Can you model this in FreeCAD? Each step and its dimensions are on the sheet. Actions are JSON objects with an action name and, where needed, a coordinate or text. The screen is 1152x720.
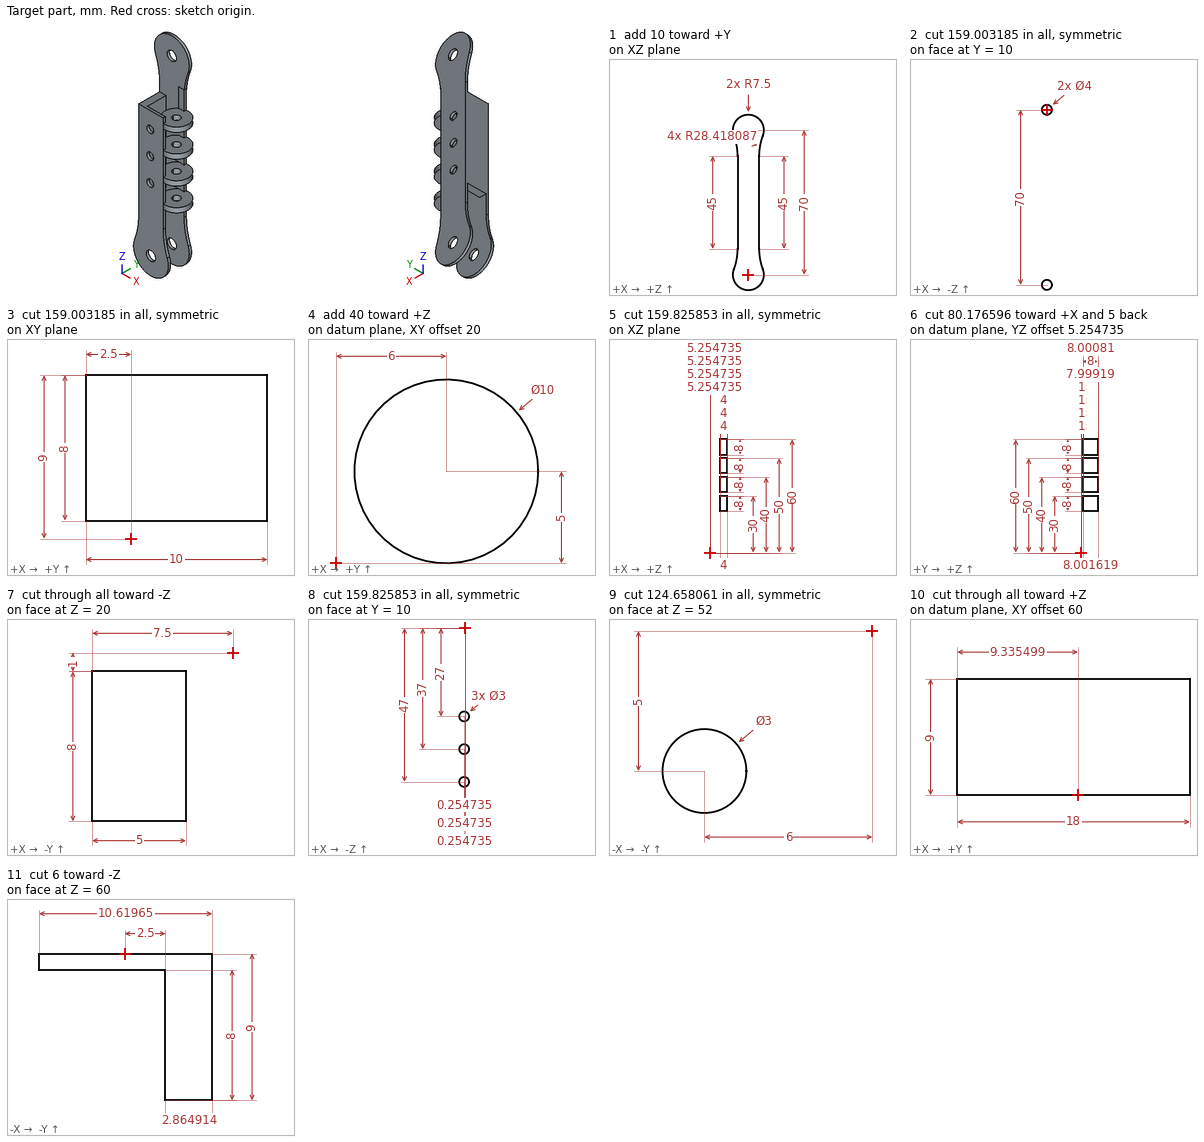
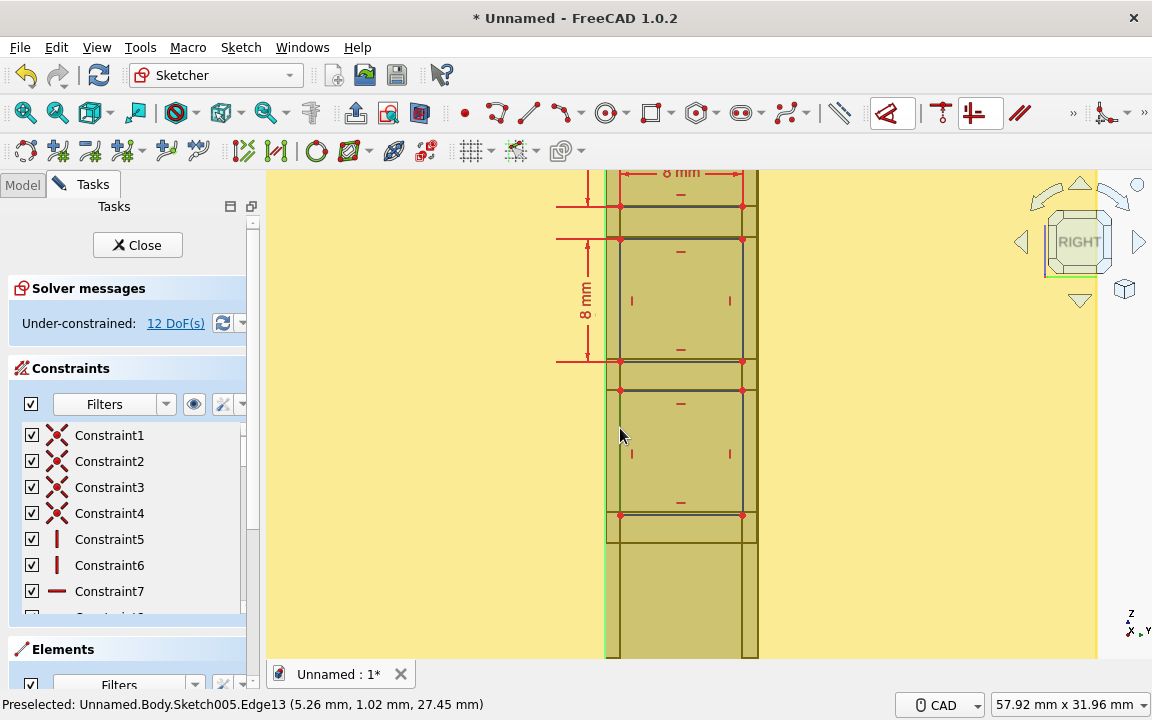
{"action": "left_click", "coordinate": [910, 114]}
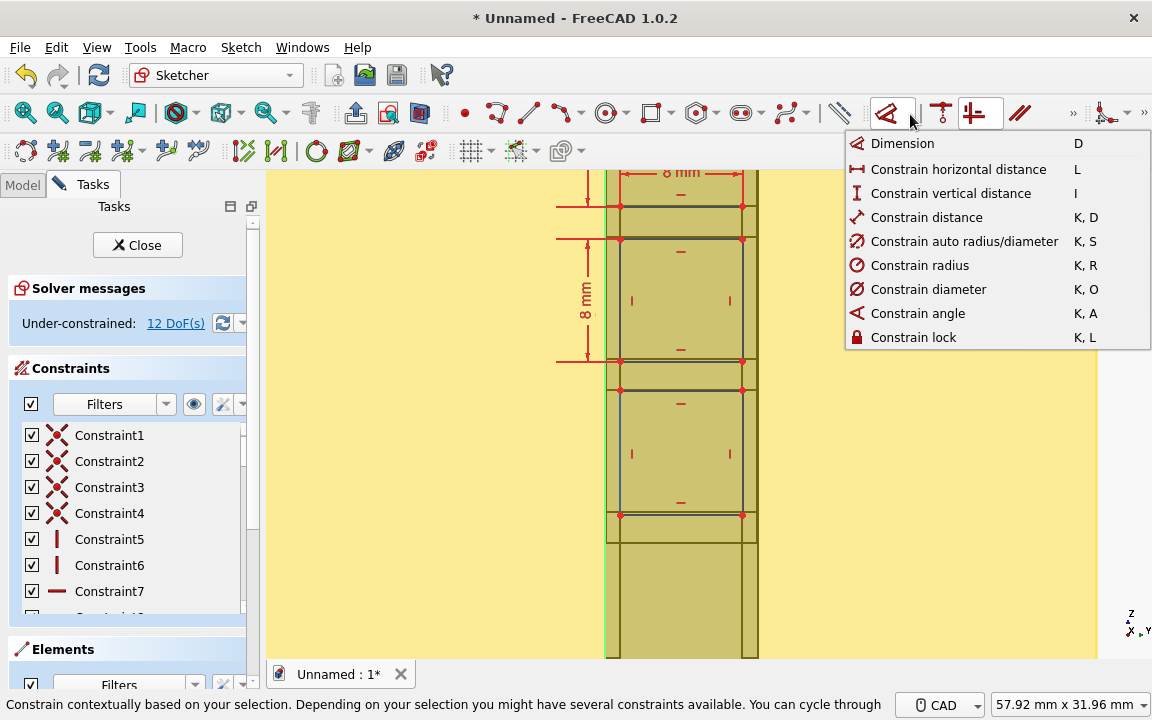
{"action": "left_click", "coordinate": [998, 193]}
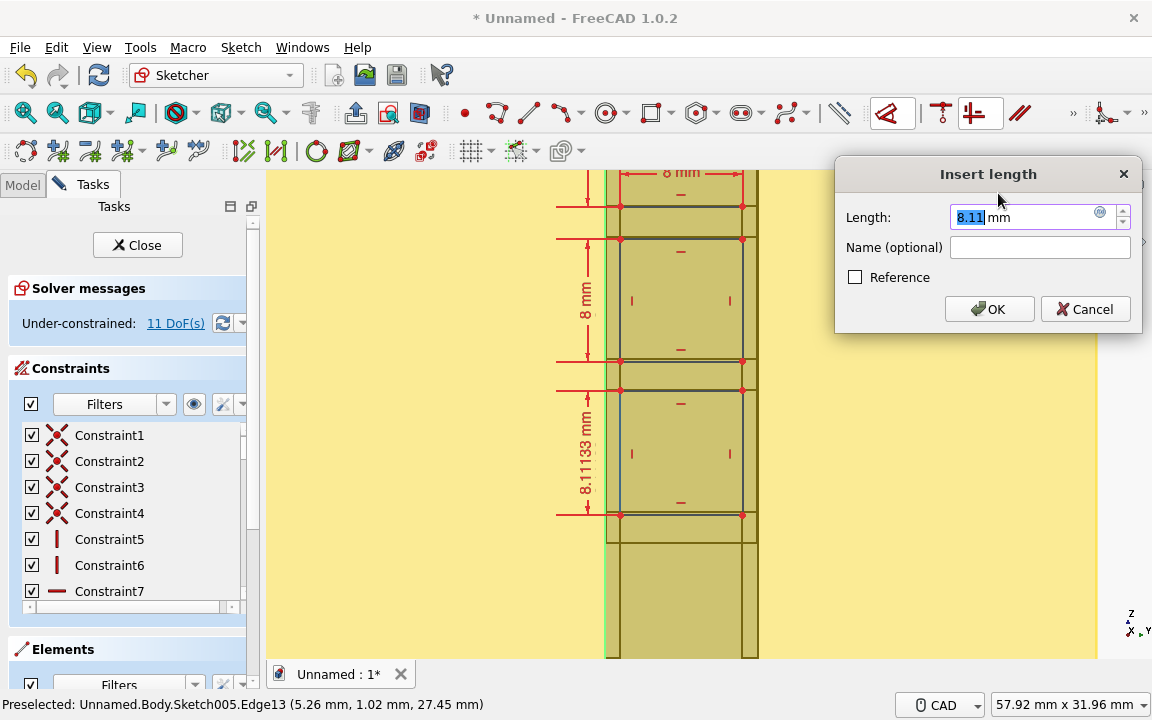
{"action": "type", "text": "8"}
{"action": "key", "text": "Return"}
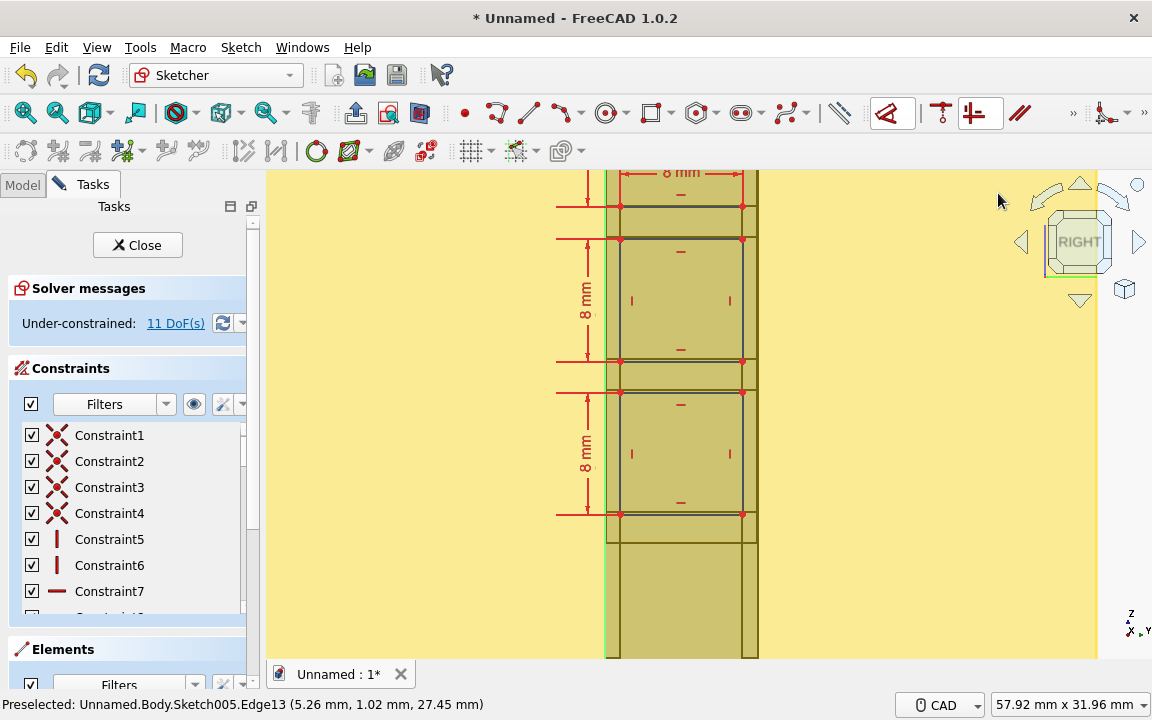
{"action": "scroll", "coordinate": [621, 429], "scroll_direction": "down", "scroll_amount": 5}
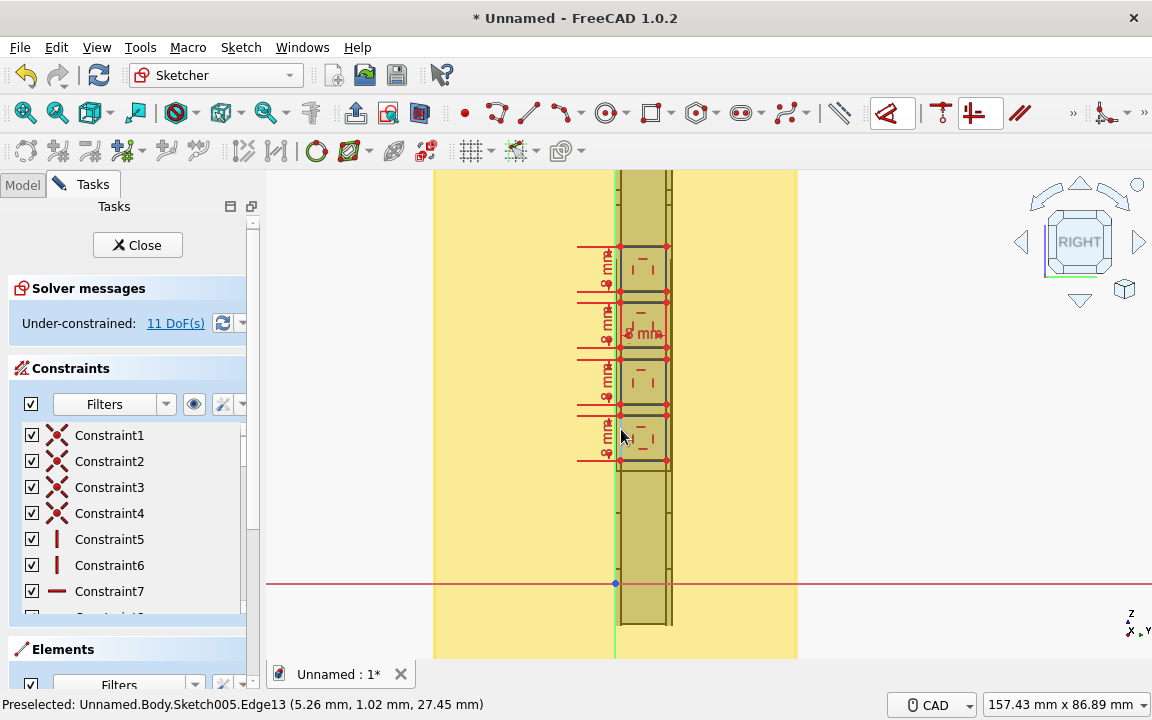
{"action": "scroll", "coordinate": [621, 247], "scroll_direction": "up", "scroll_amount": 10}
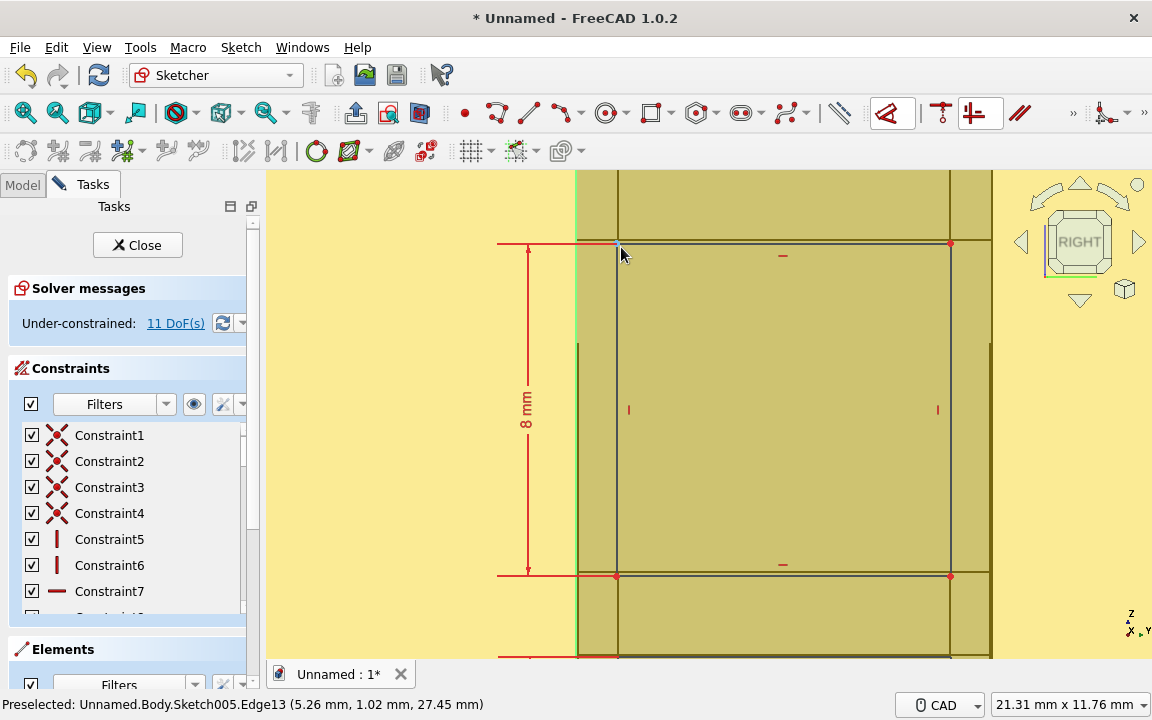
{"action": "left_click", "coordinate": [617, 244]}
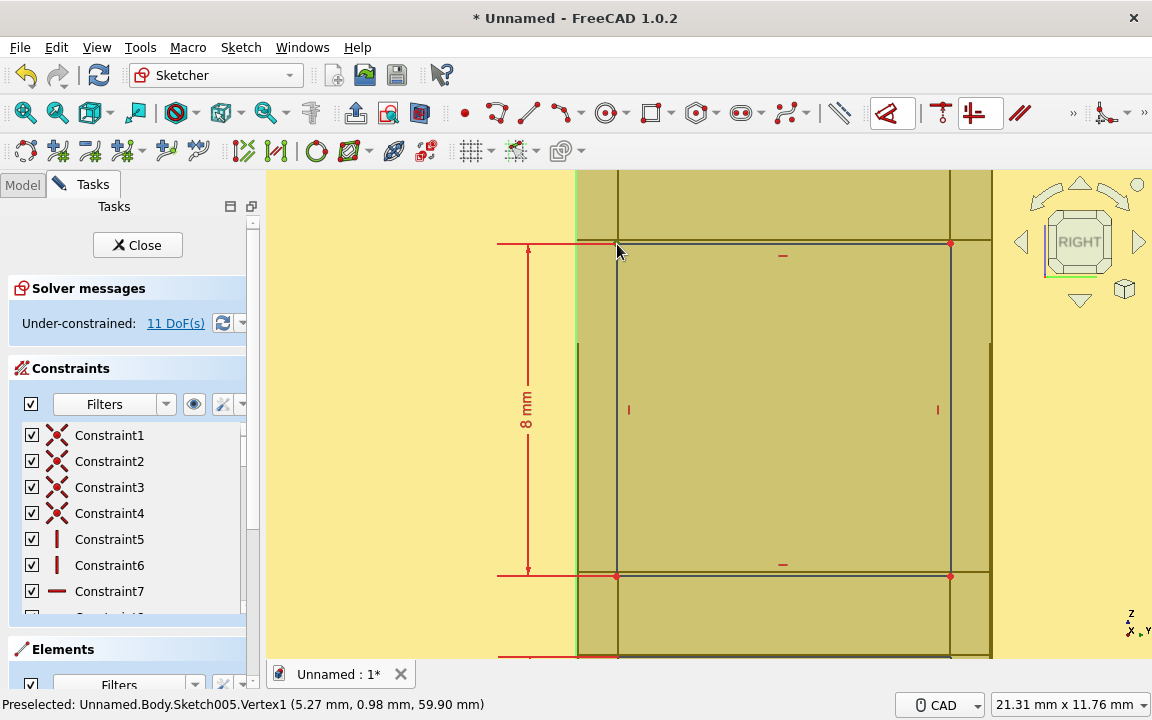
{"action": "key", "text": "l"}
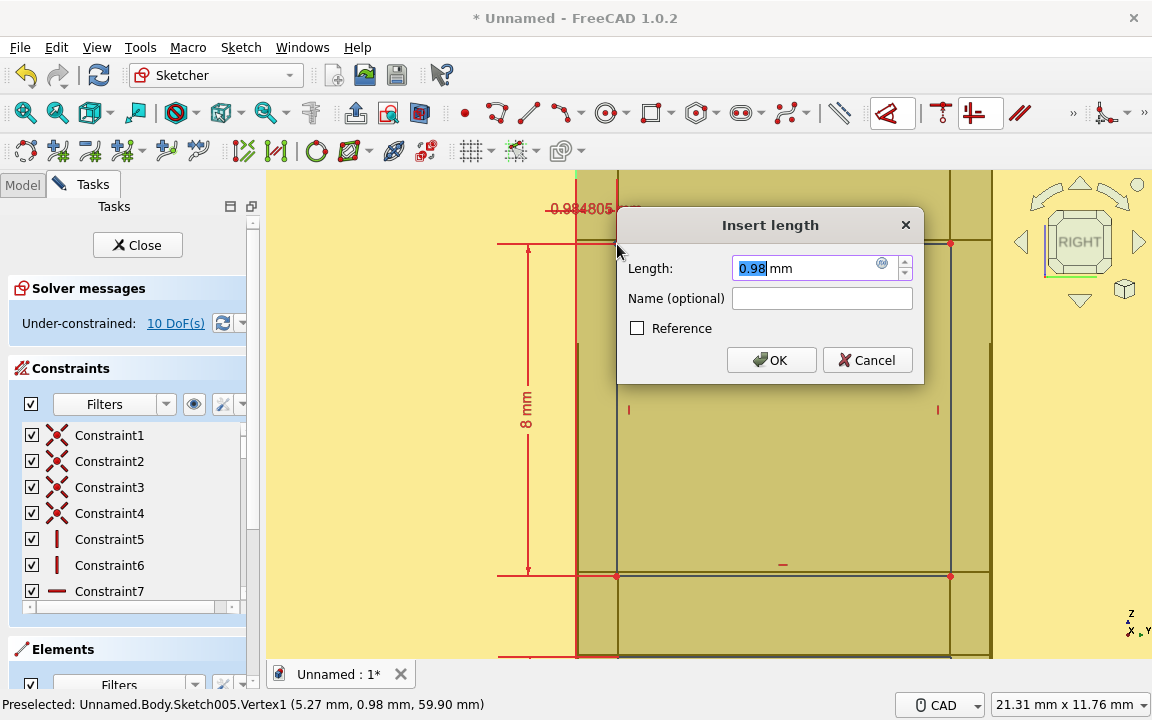
{"action": "type", "text": "1"}
{"action": "key", "text": "Return"}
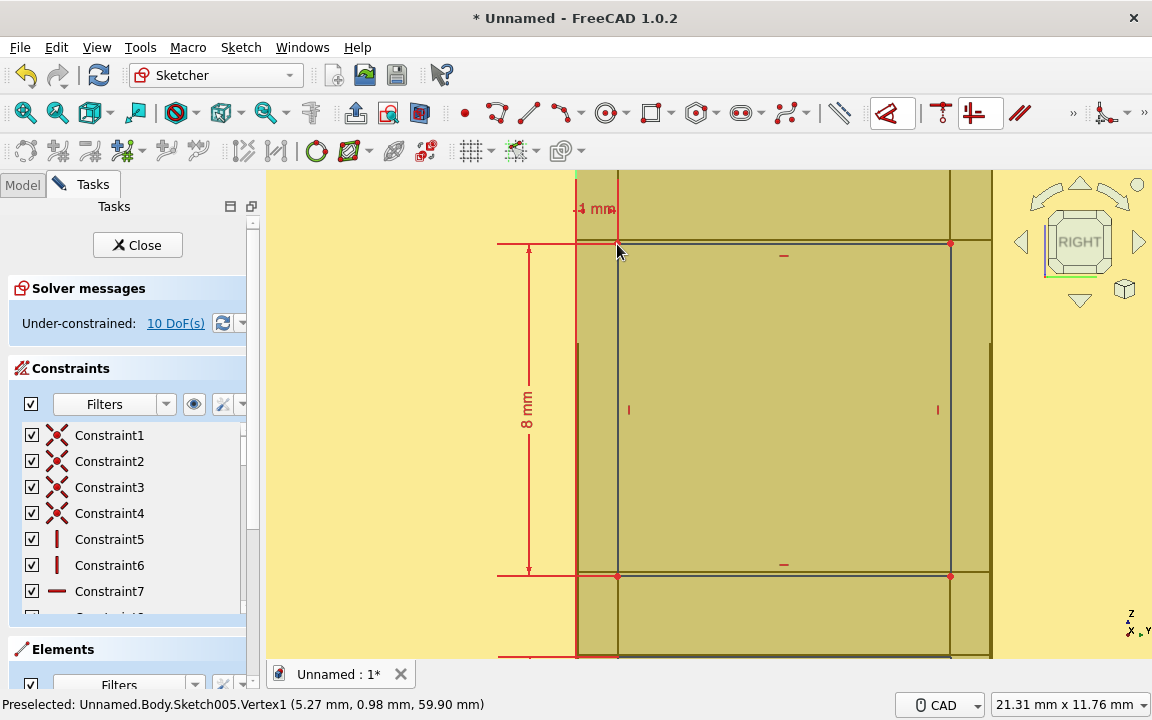
{"action": "scroll", "coordinate": [621, 247], "scroll_direction": "down", "scroll_amount": 10}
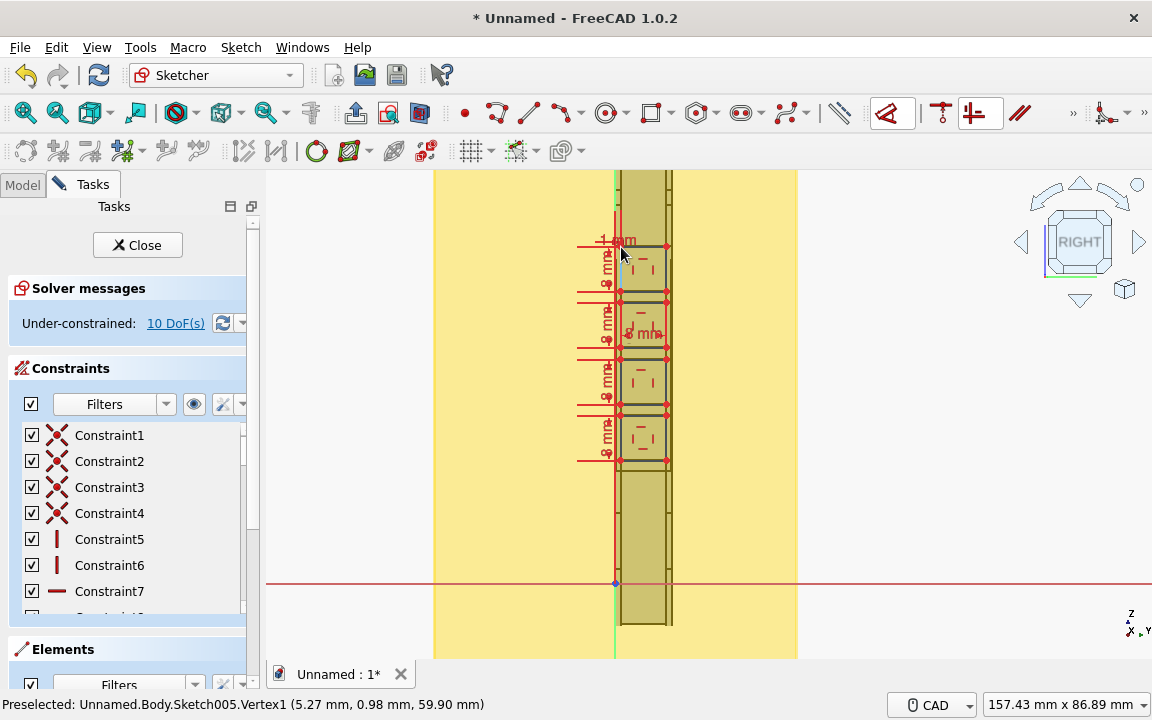
{"action": "scroll", "coordinate": [621, 303], "scroll_direction": "up", "scroll_amount": 10}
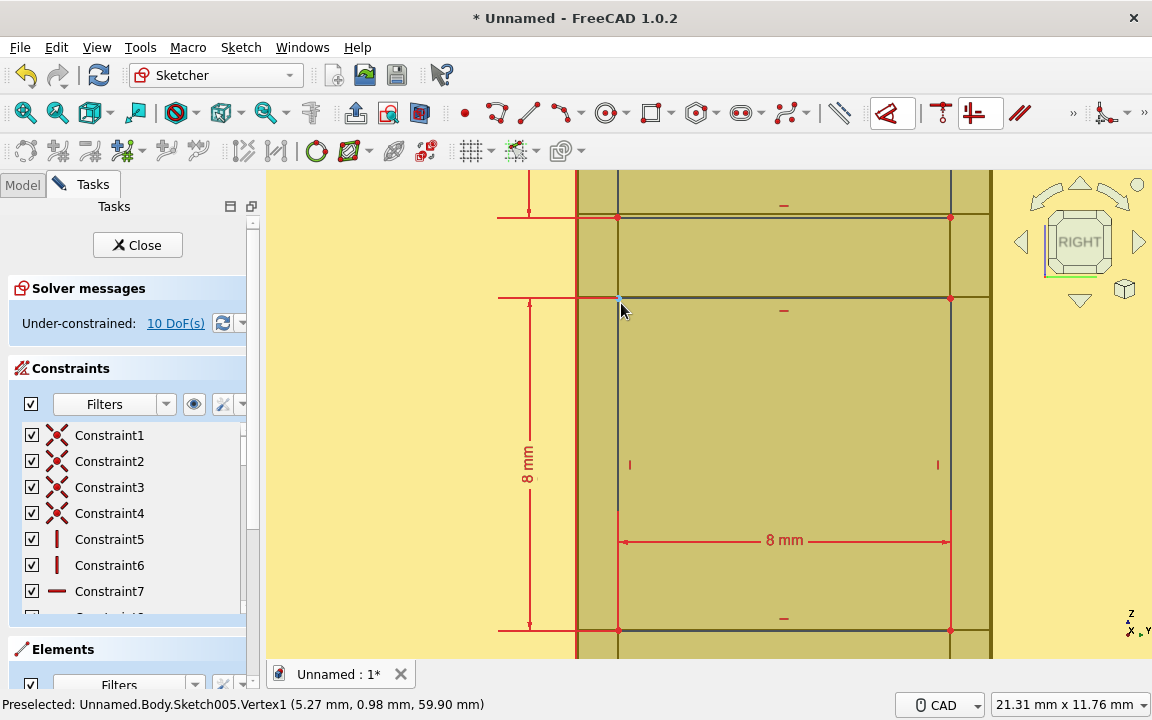
{"action": "left_click", "coordinate": [618, 298]}